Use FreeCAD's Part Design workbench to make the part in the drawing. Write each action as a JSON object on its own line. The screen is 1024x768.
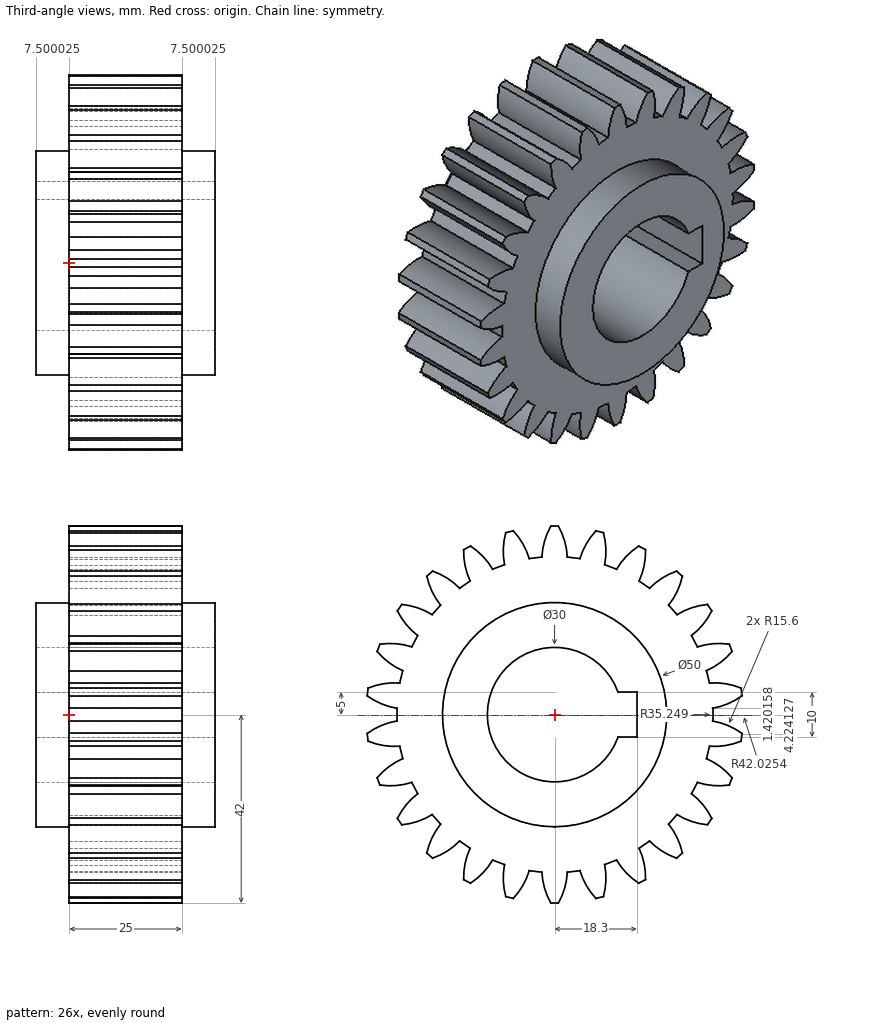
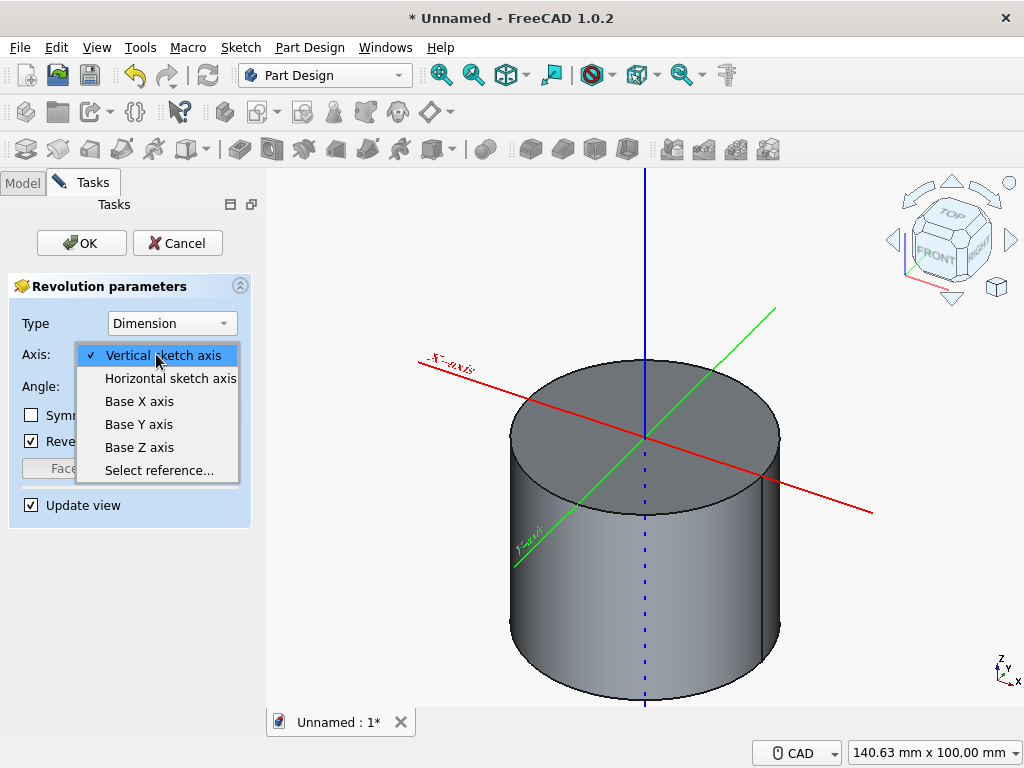
{"action": "left_click", "coordinate": [156, 378]}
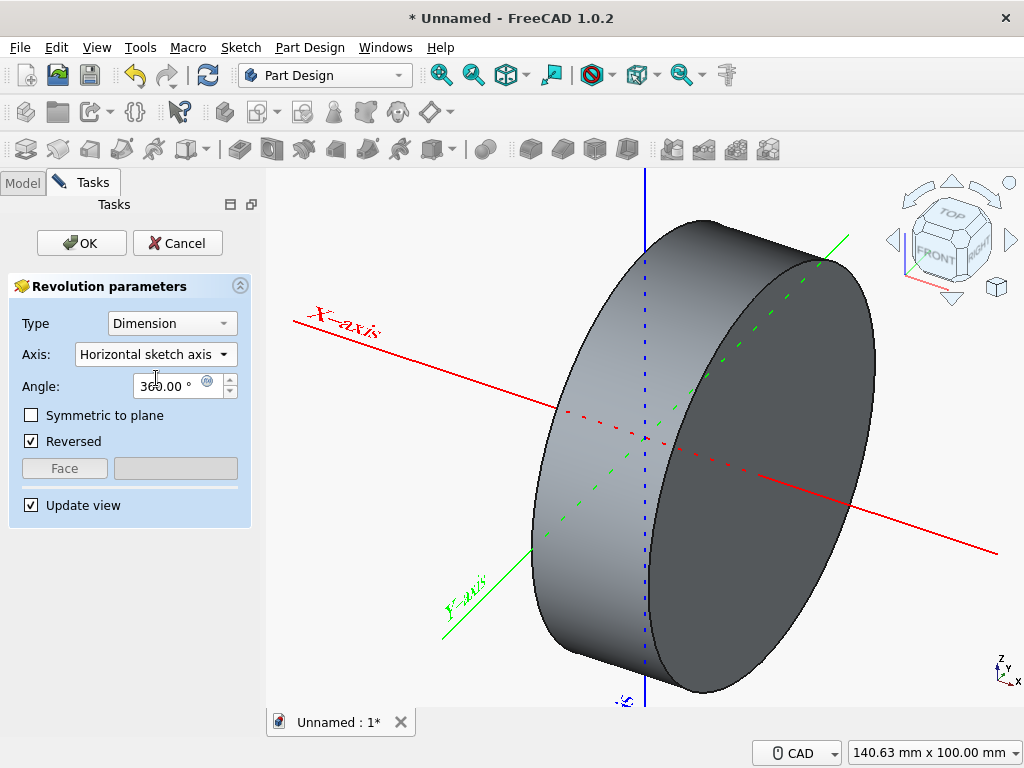
{"action": "left_click", "coordinate": [82, 243]}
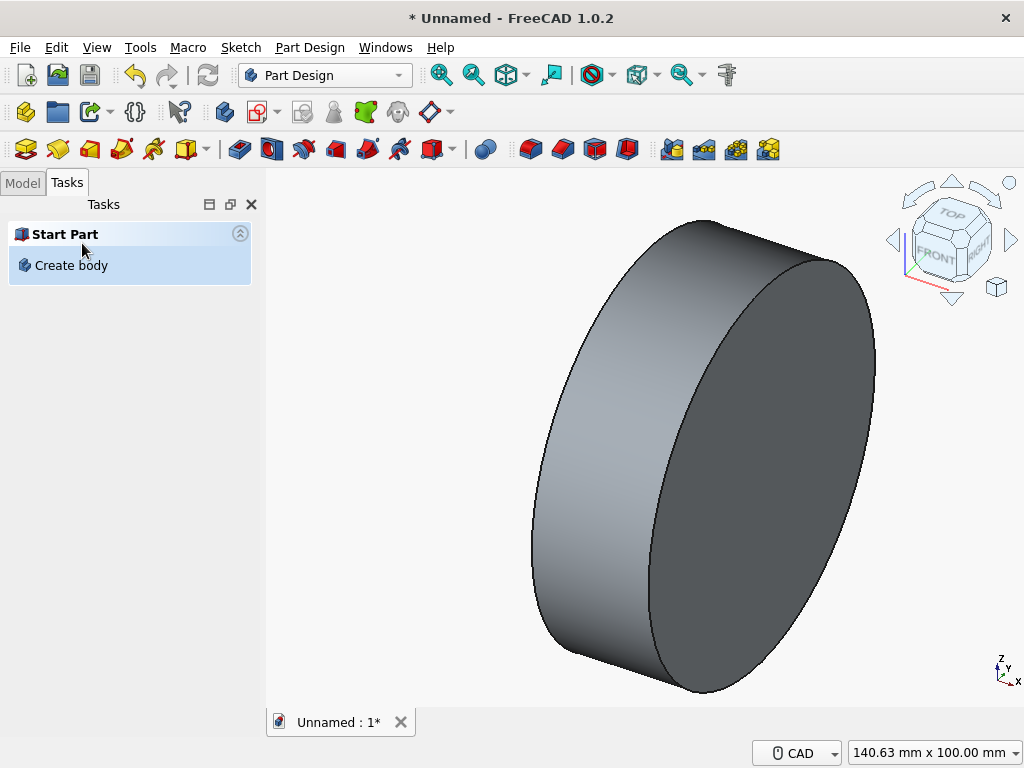
{"action": "left_click", "coordinate": [442, 76]}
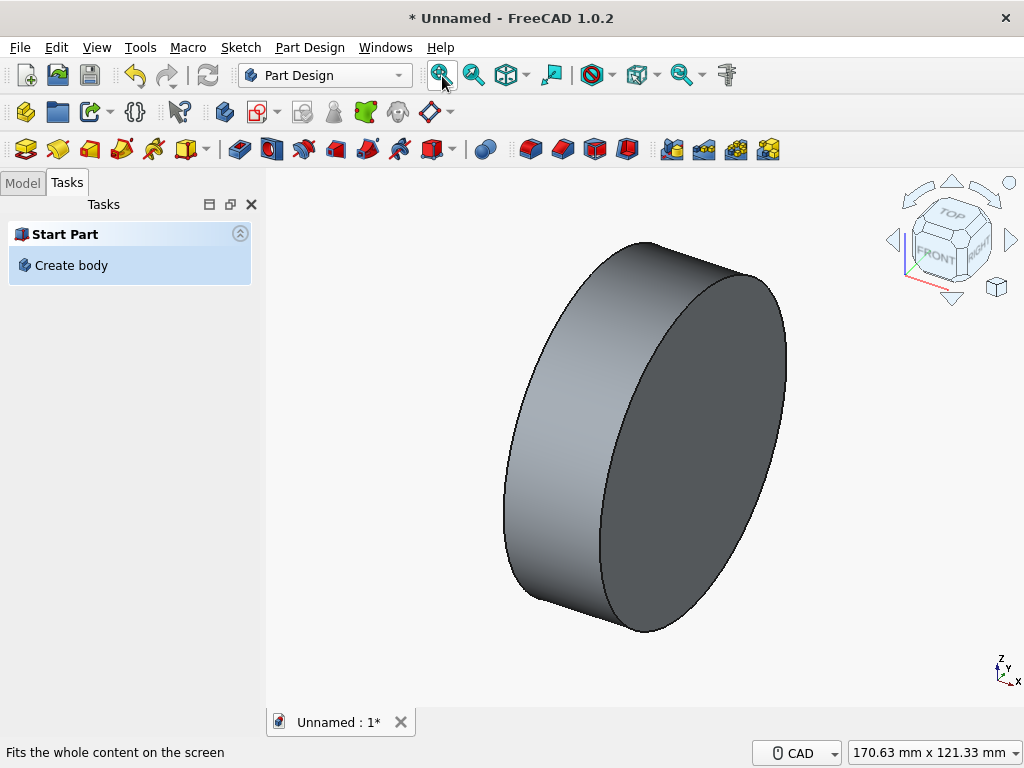
{"action": "key", "text": "6"}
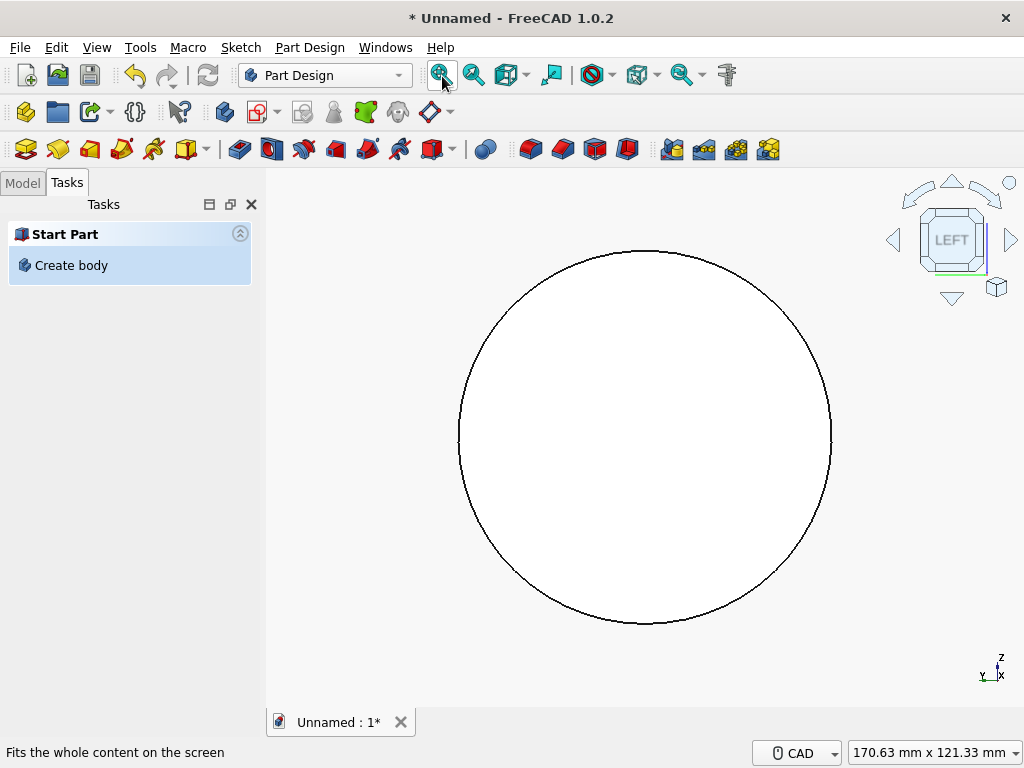
{"action": "left_click", "coordinate": [645, 436]}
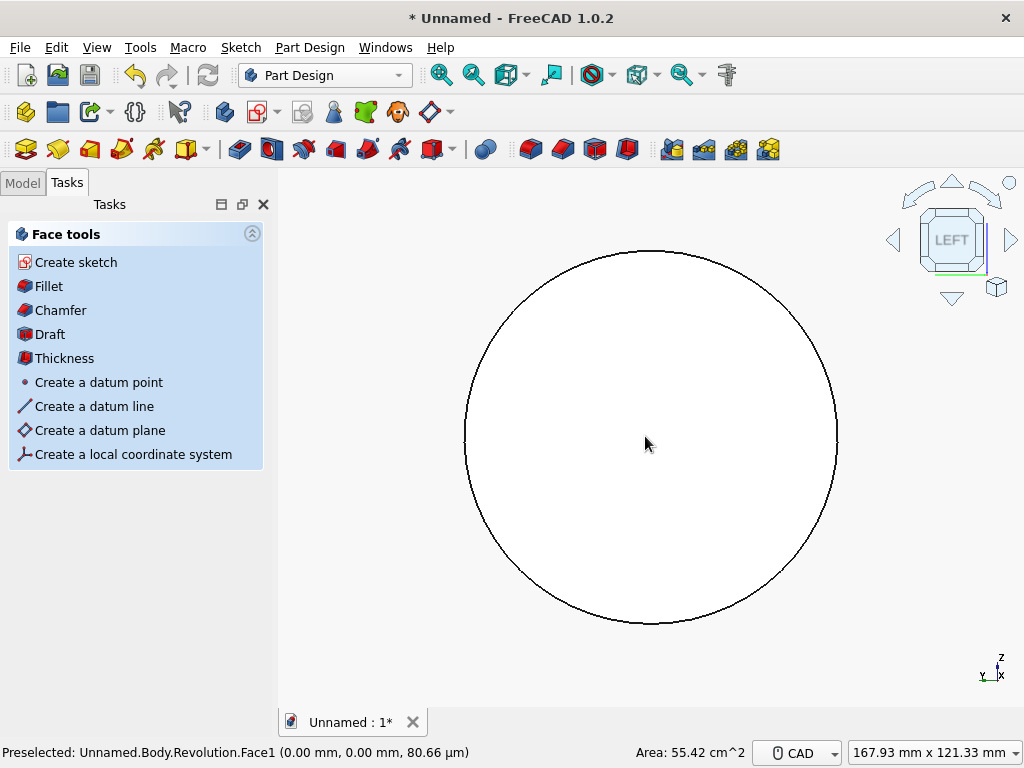
{"action": "left_click", "coordinate": [258, 112]}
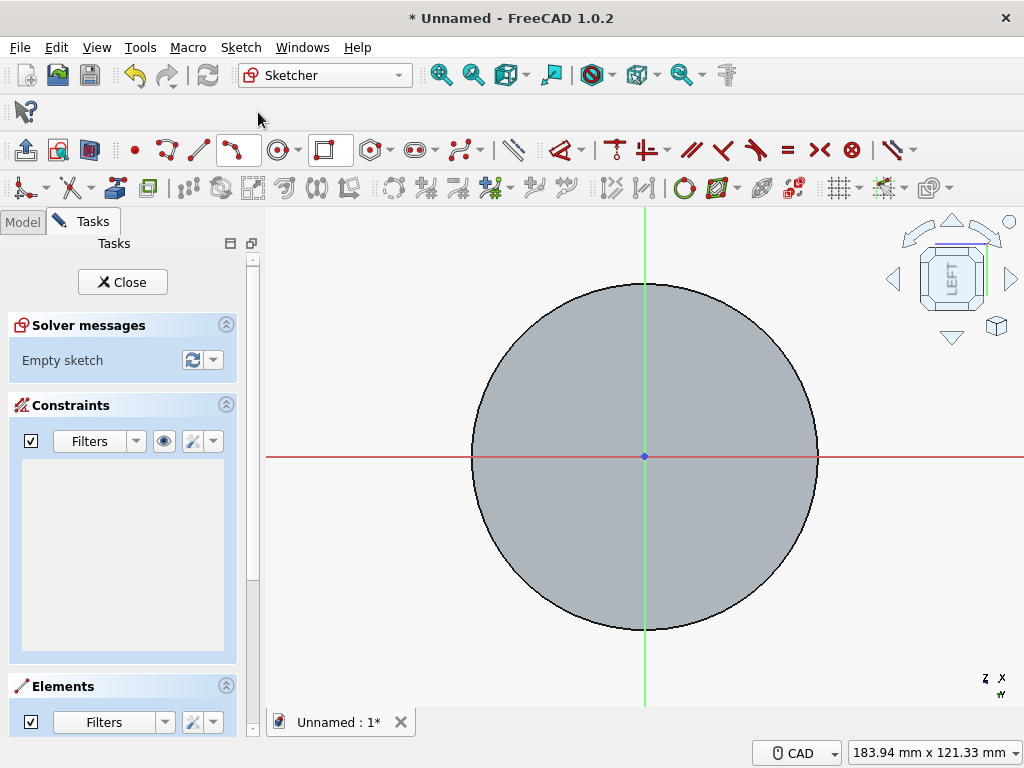
{"action": "scroll", "coordinate": [652, 632], "scroll_direction": "up", "scroll_amount": 12}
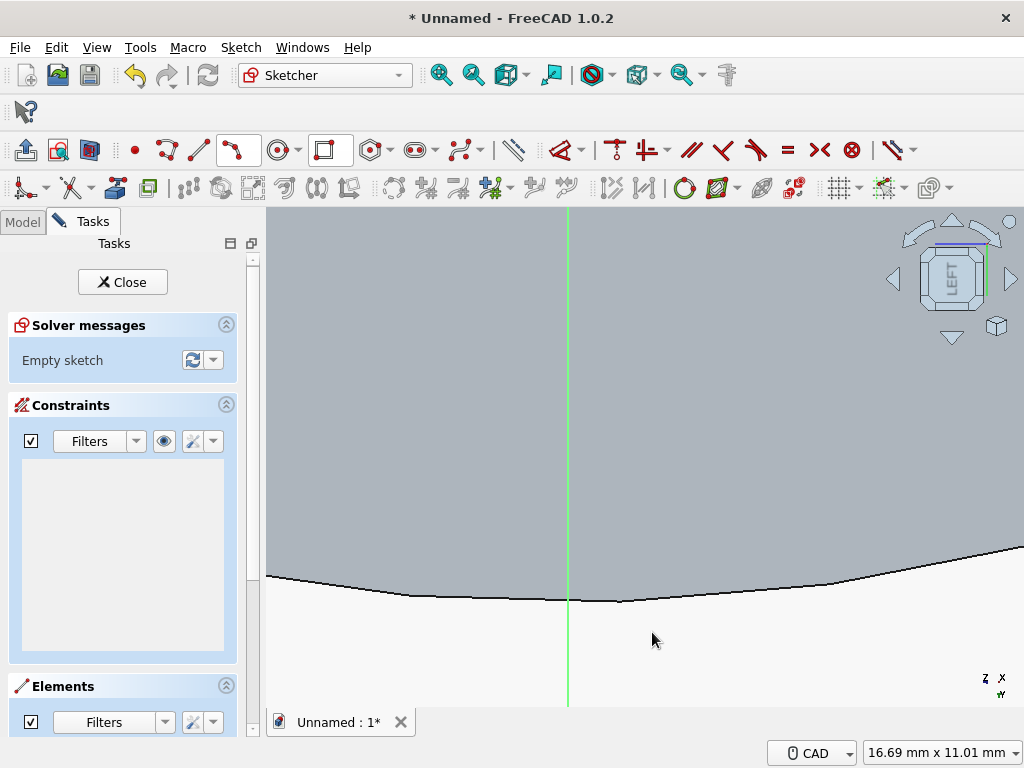
{"action": "left_click", "coordinate": [232, 150]}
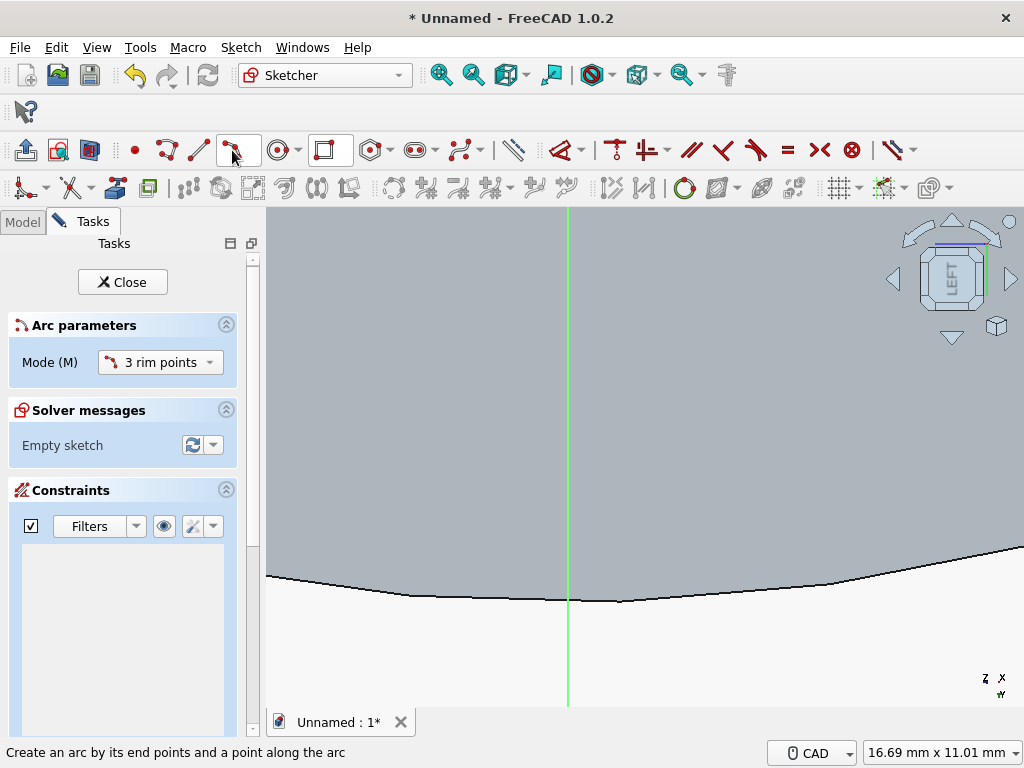
{"action": "left_click", "coordinate": [504, 294]}
{"action": "left_click", "coordinate": [633, 294]}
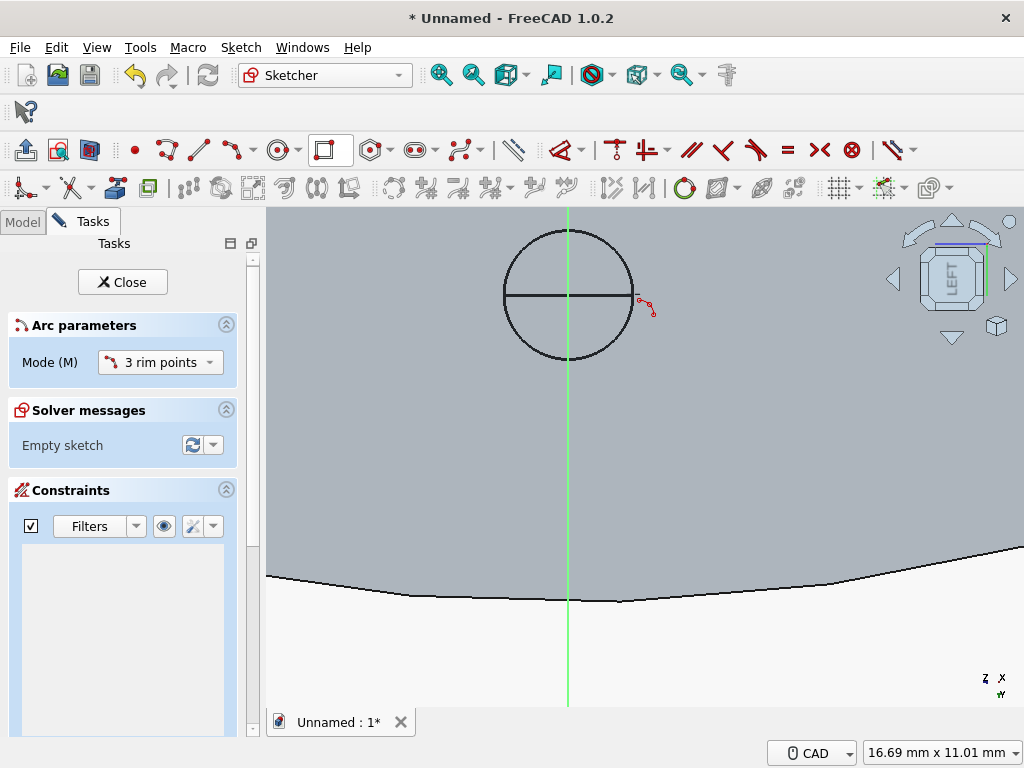
{"action": "scroll", "coordinate": [555, 296], "scroll_direction": "up", "scroll_amount": 13}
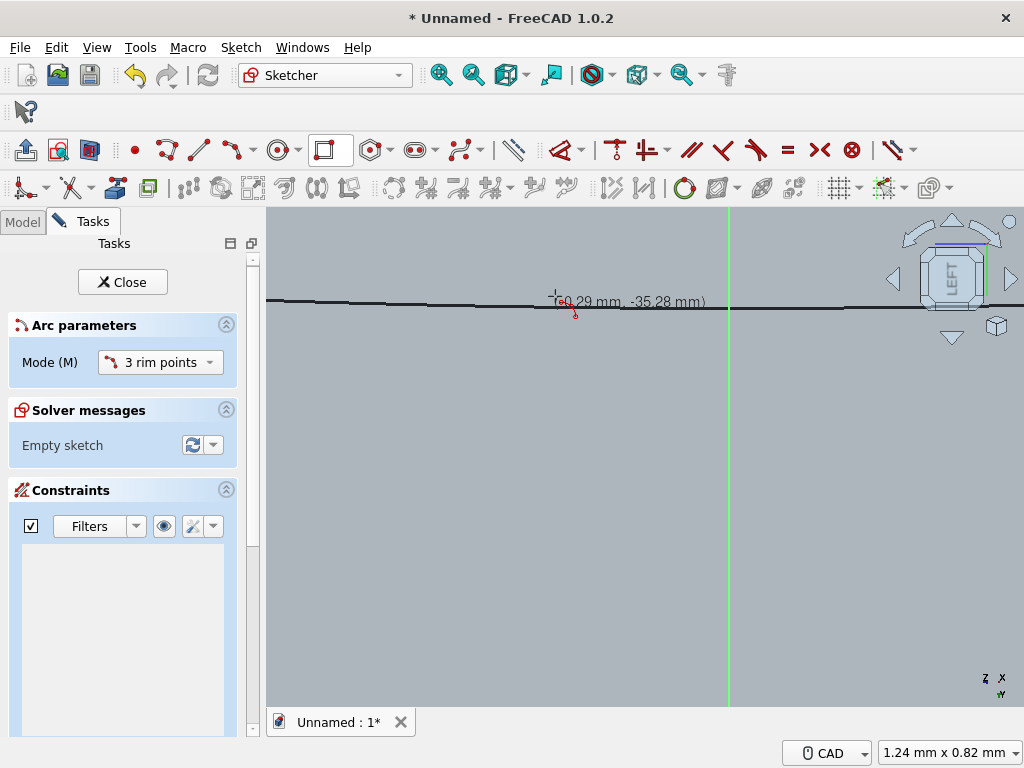
{"action": "left_click", "coordinate": [555, 288]}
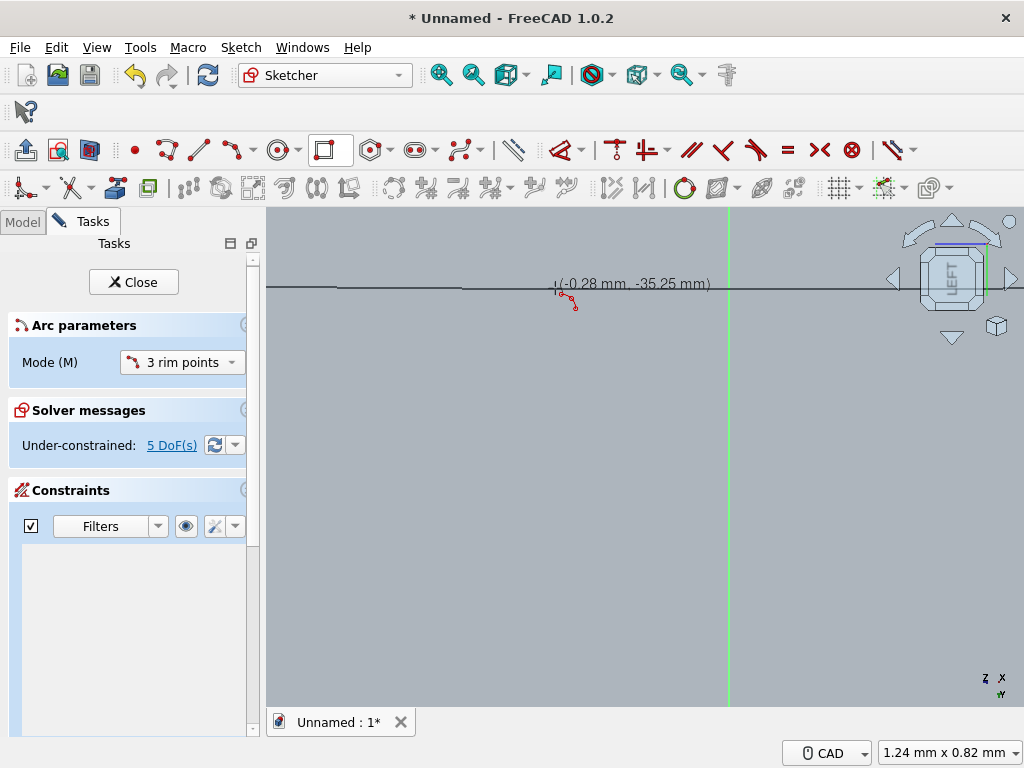
{"action": "scroll", "coordinate": [564, 305], "scroll_direction": "down", "scroll_amount": 13}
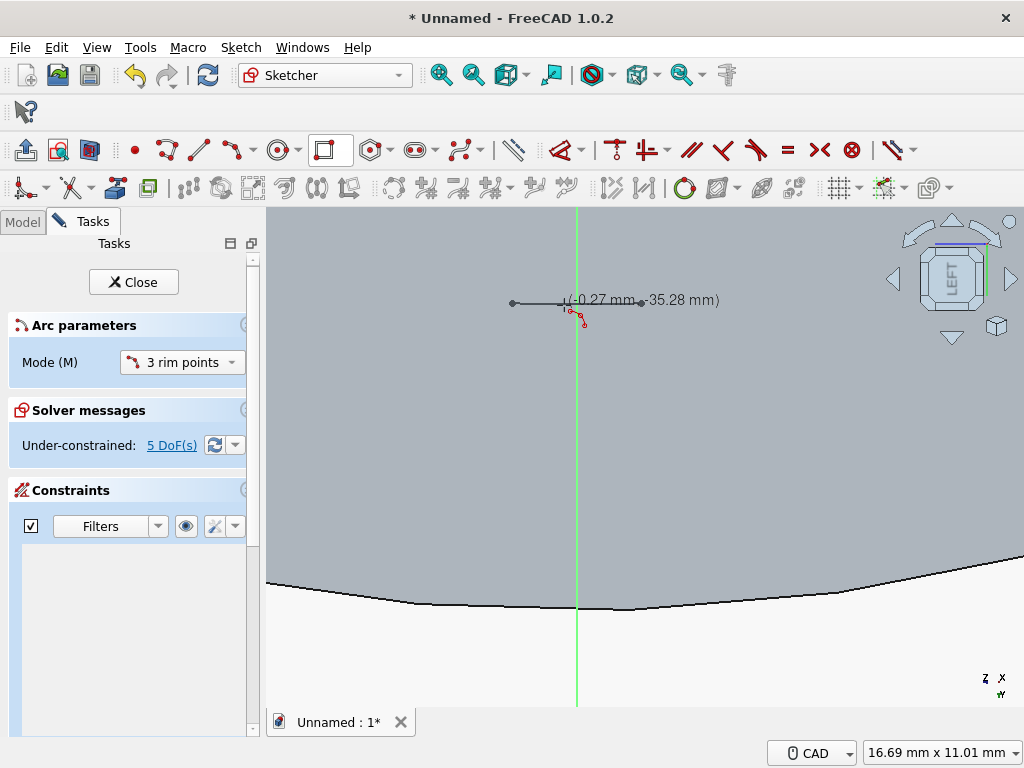
{"action": "left_click", "coordinate": [641, 303]}
{"action": "left_click", "coordinate": [769, 602]}
{"action": "left_click", "coordinate": [687, 460]}